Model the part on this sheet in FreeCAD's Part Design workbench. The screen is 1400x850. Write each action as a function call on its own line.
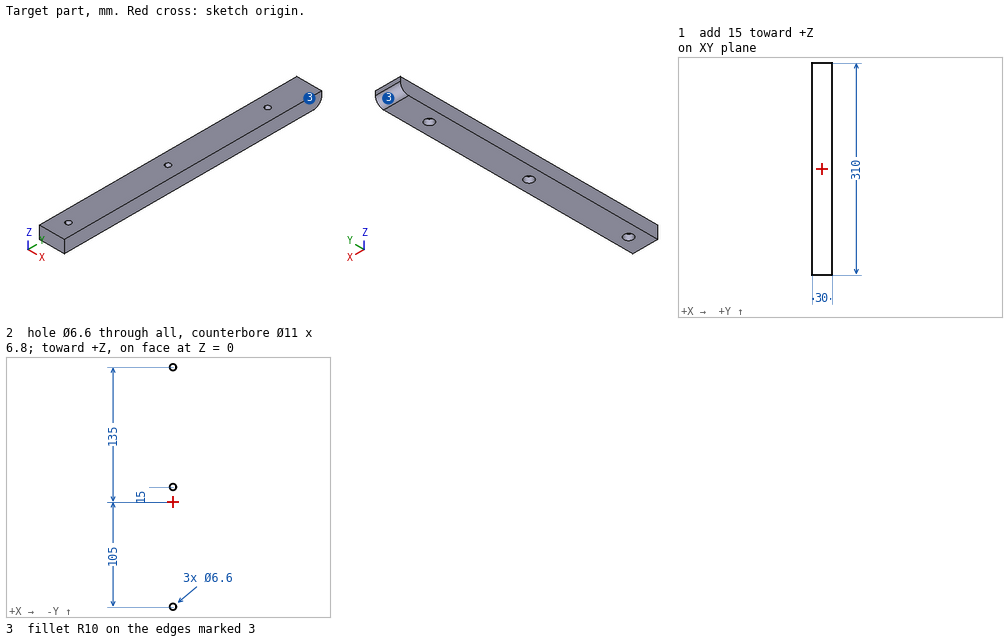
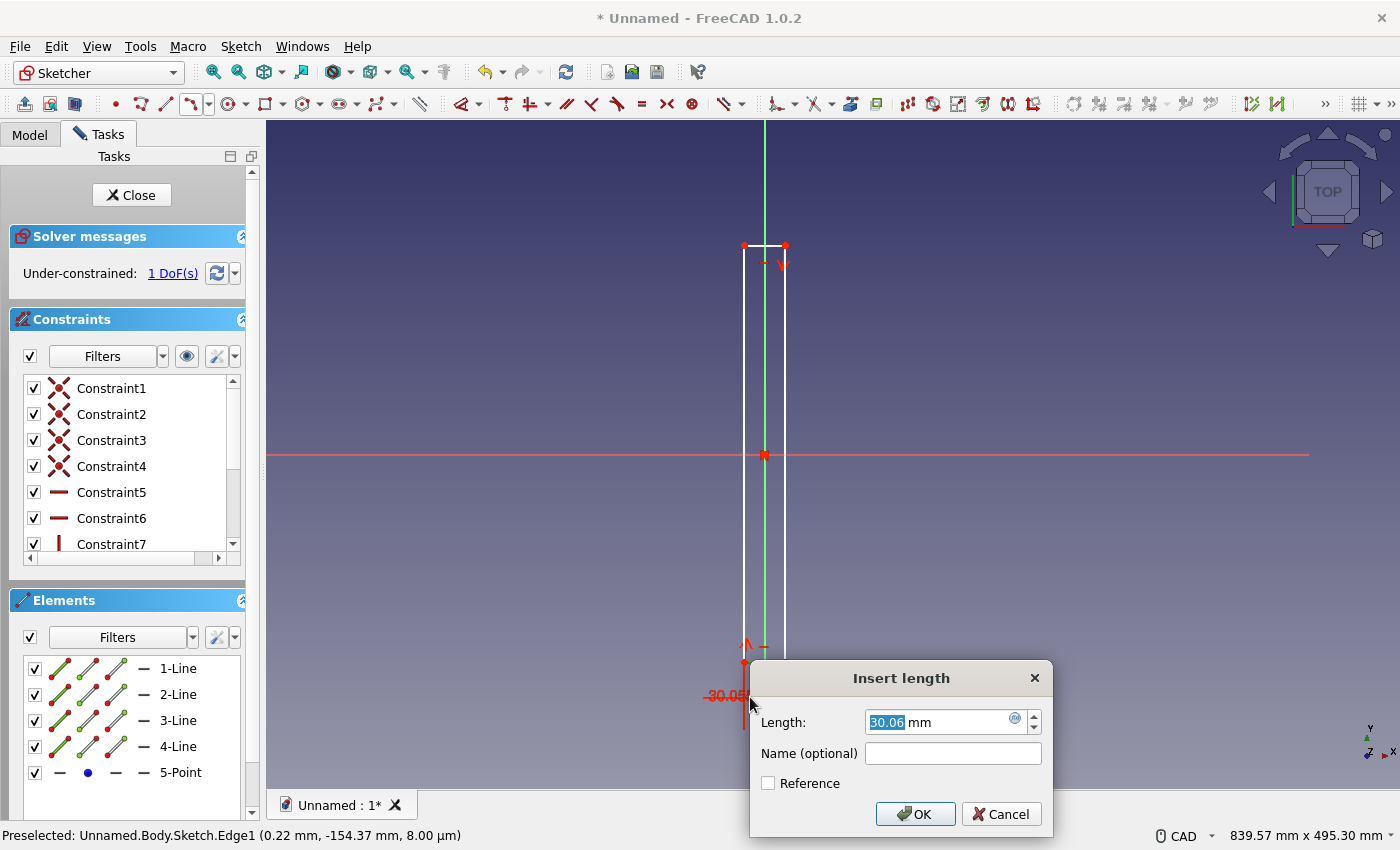
text(30)
key(Return)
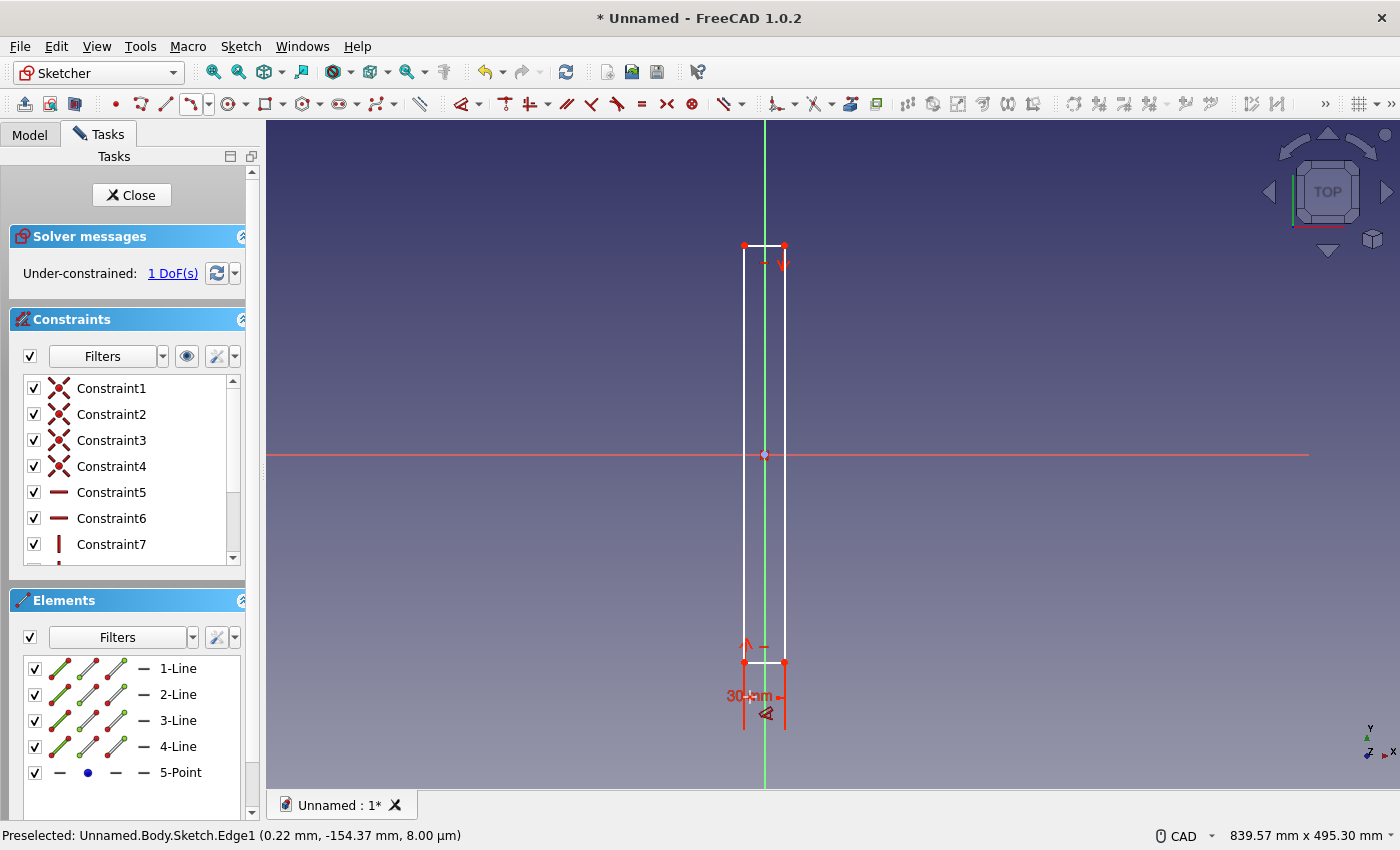
click(785, 538)
click(819, 359)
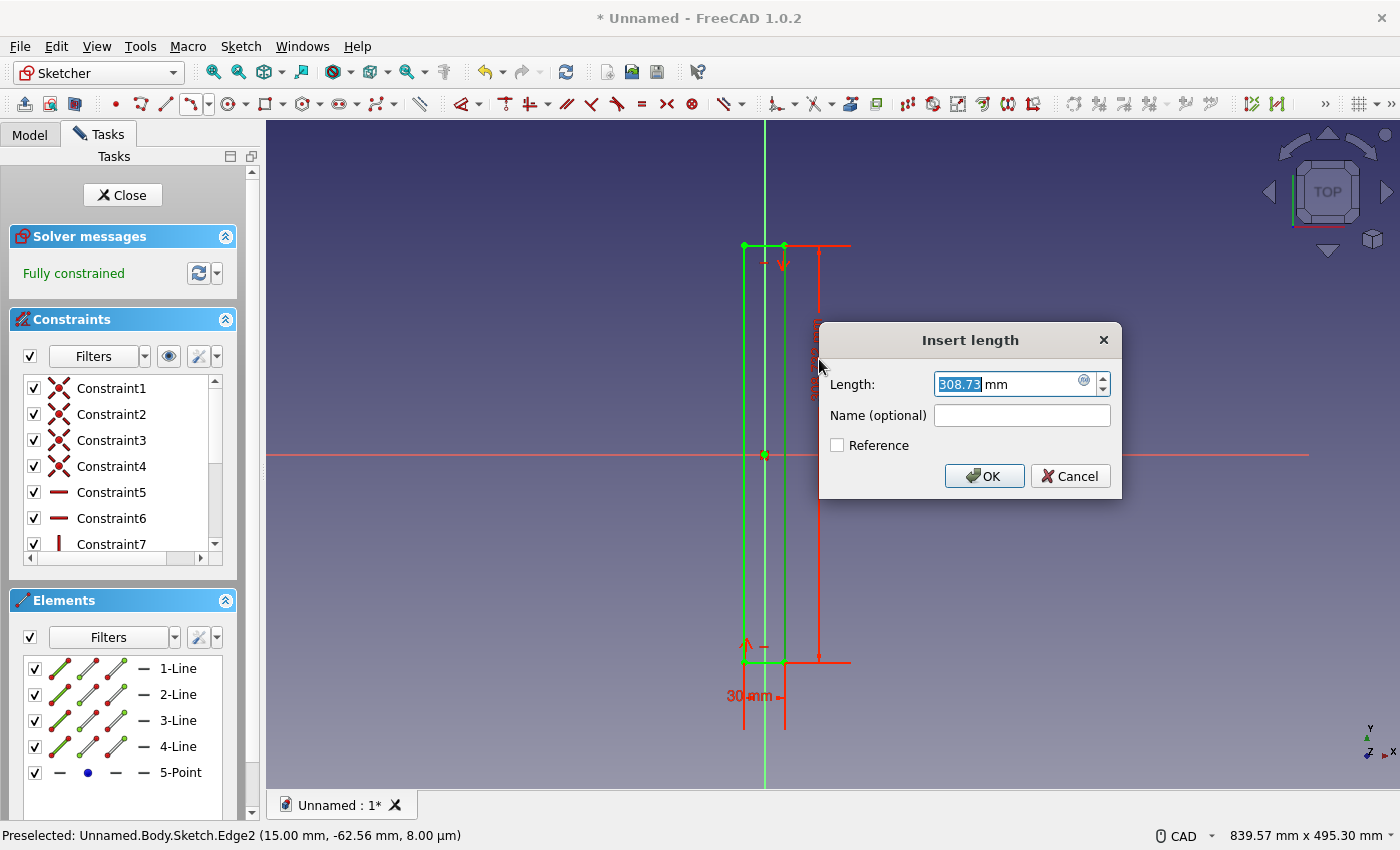
text(310)
key(Return)
key(Escape)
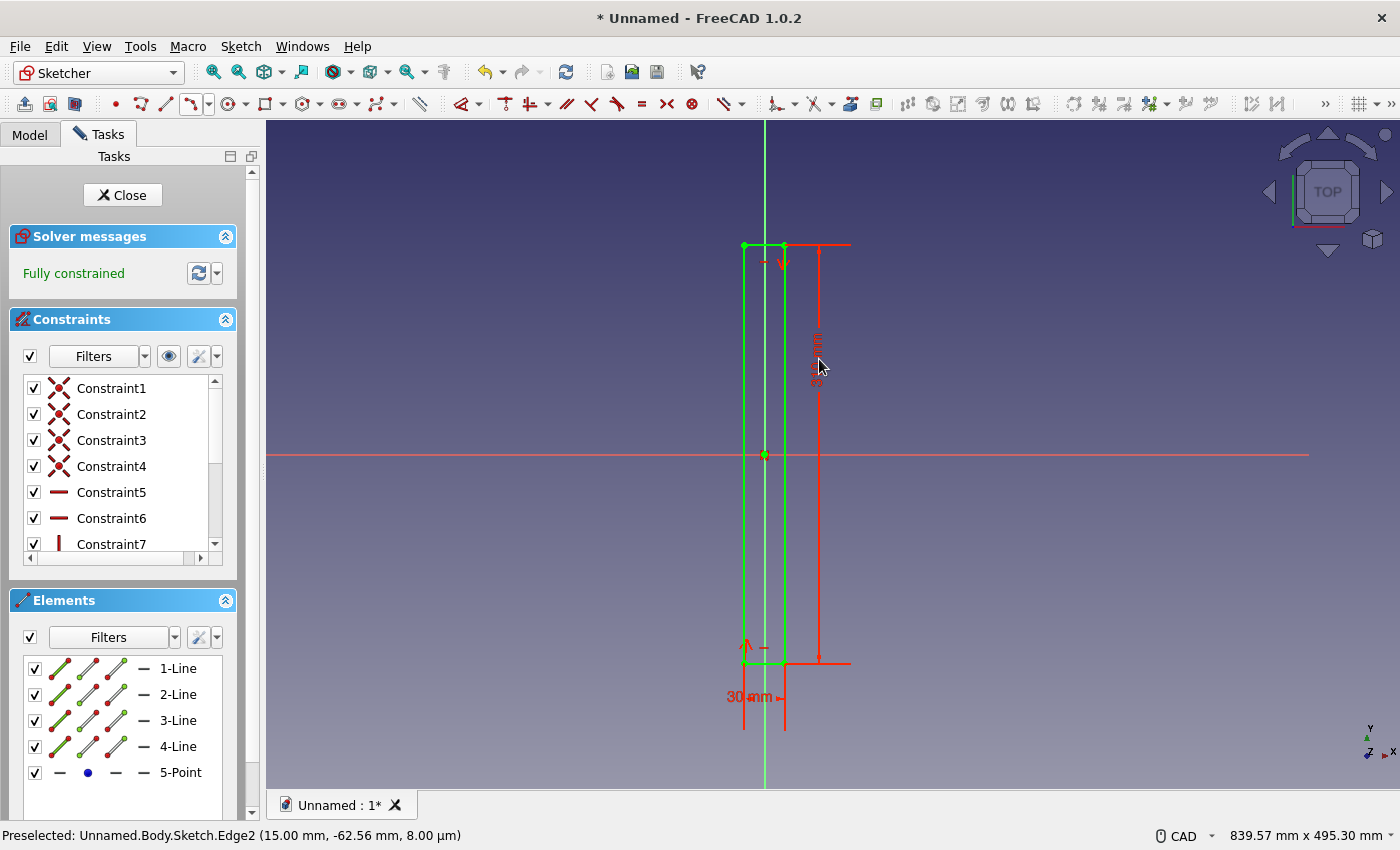
click(123, 195)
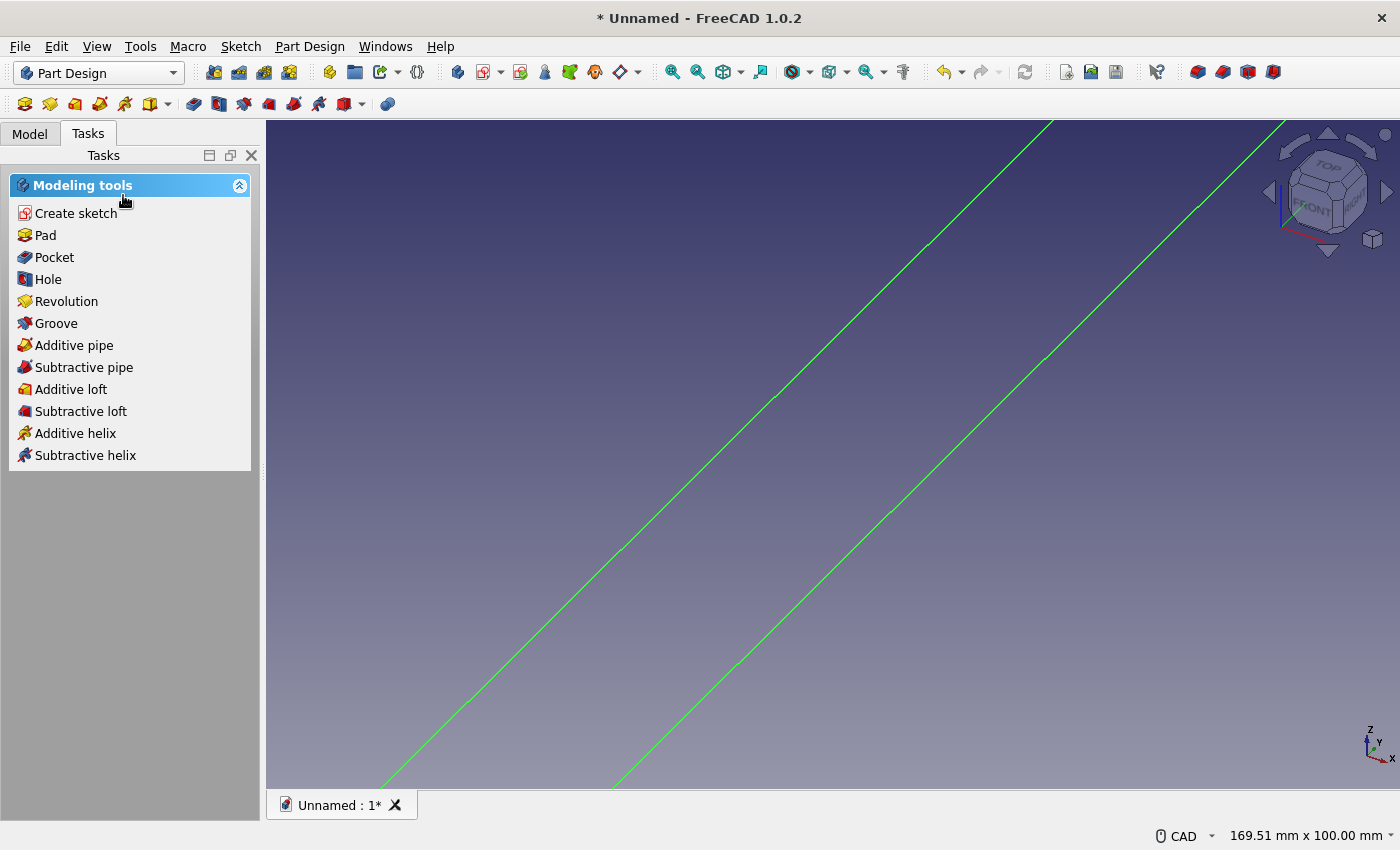
click(25, 104)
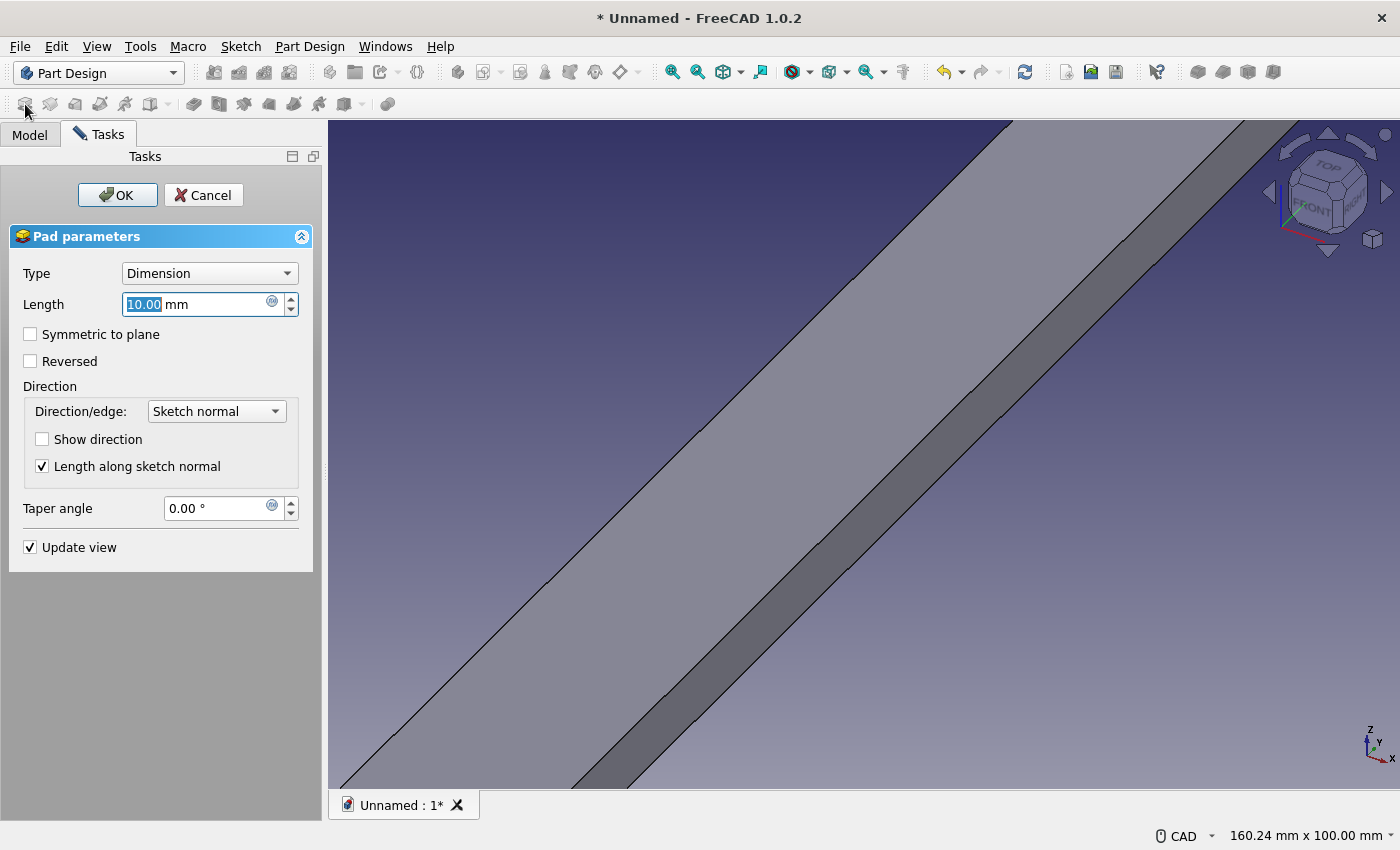
text(15)
key(Tab)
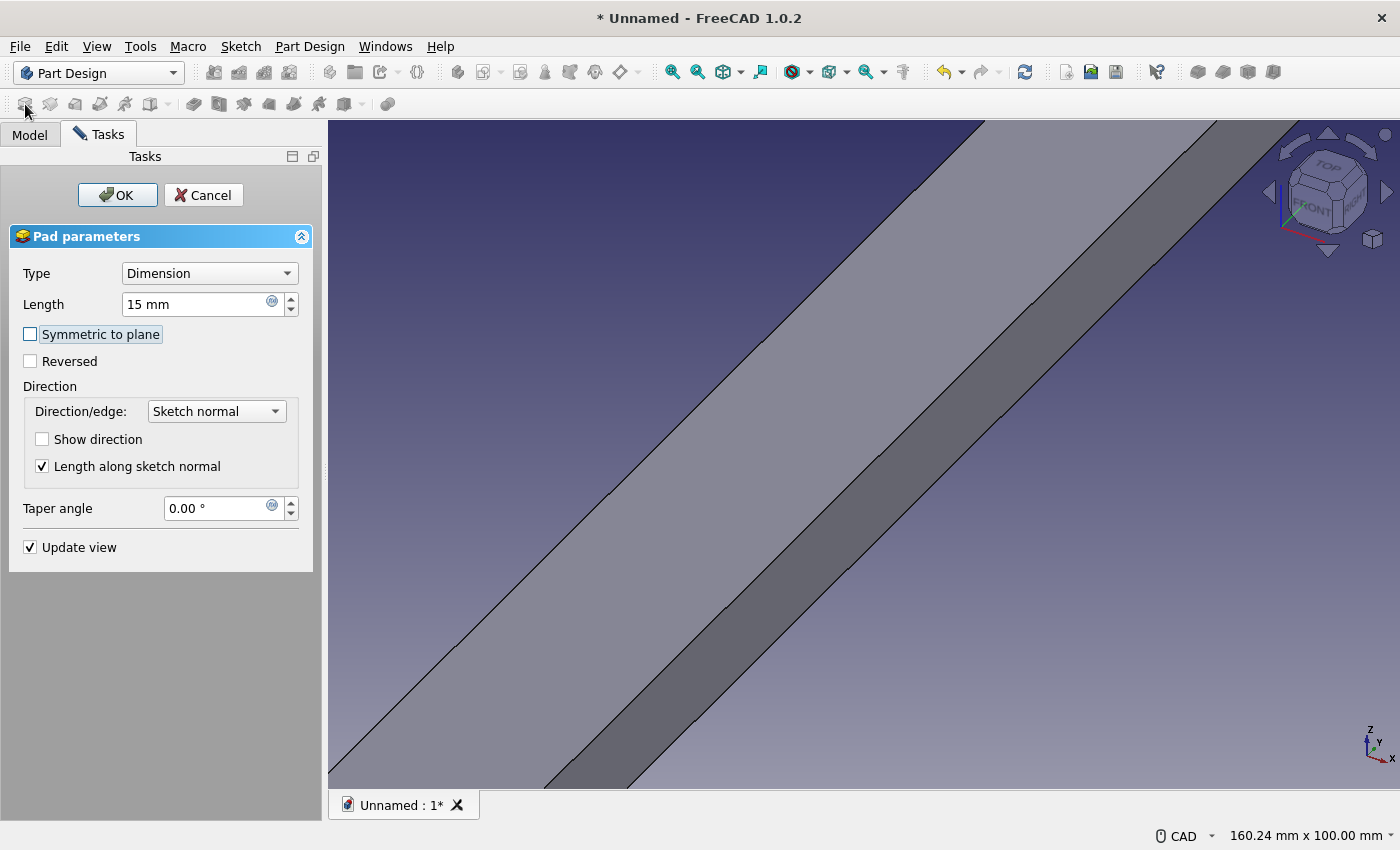
click(118, 195)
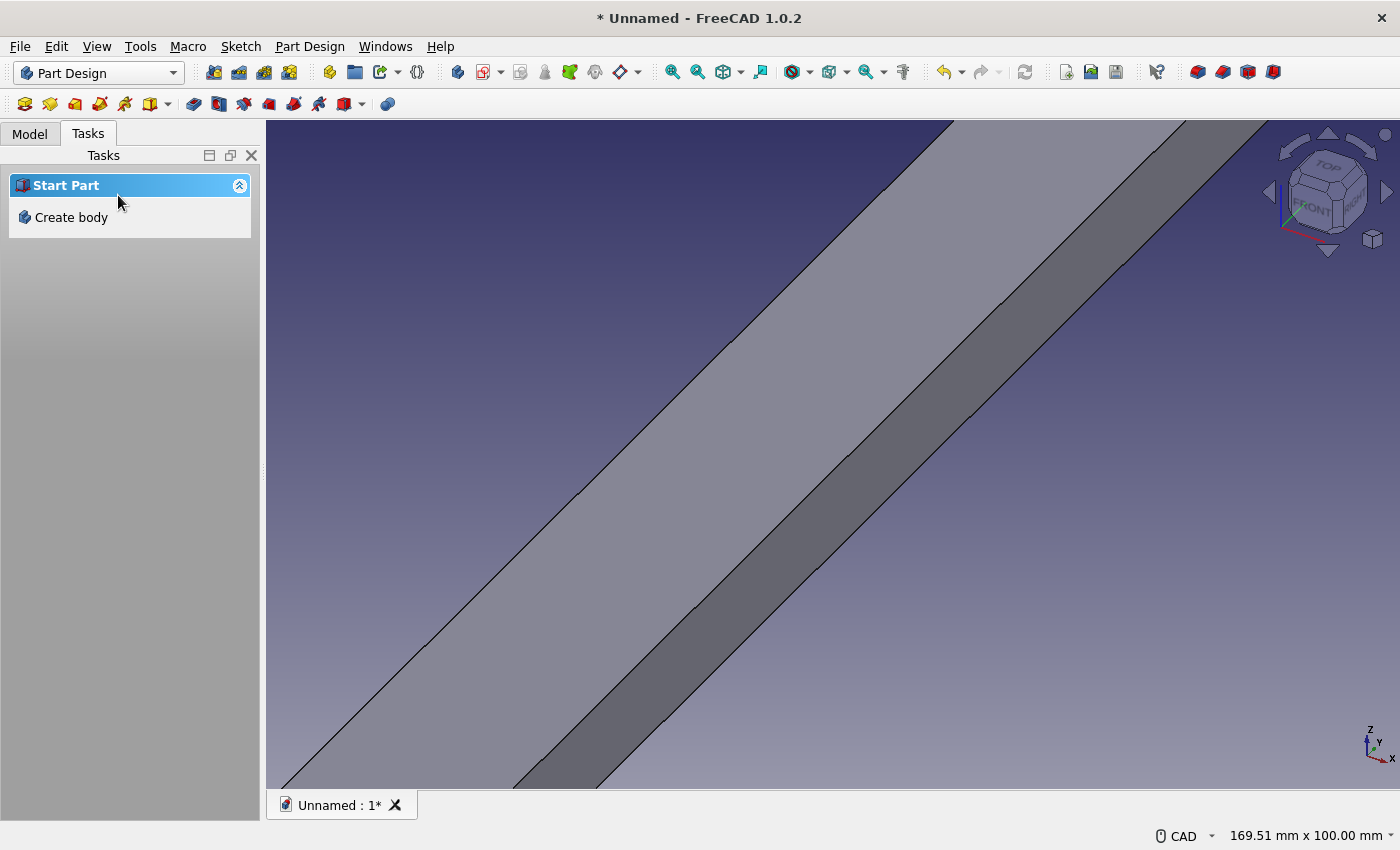
click(673, 72)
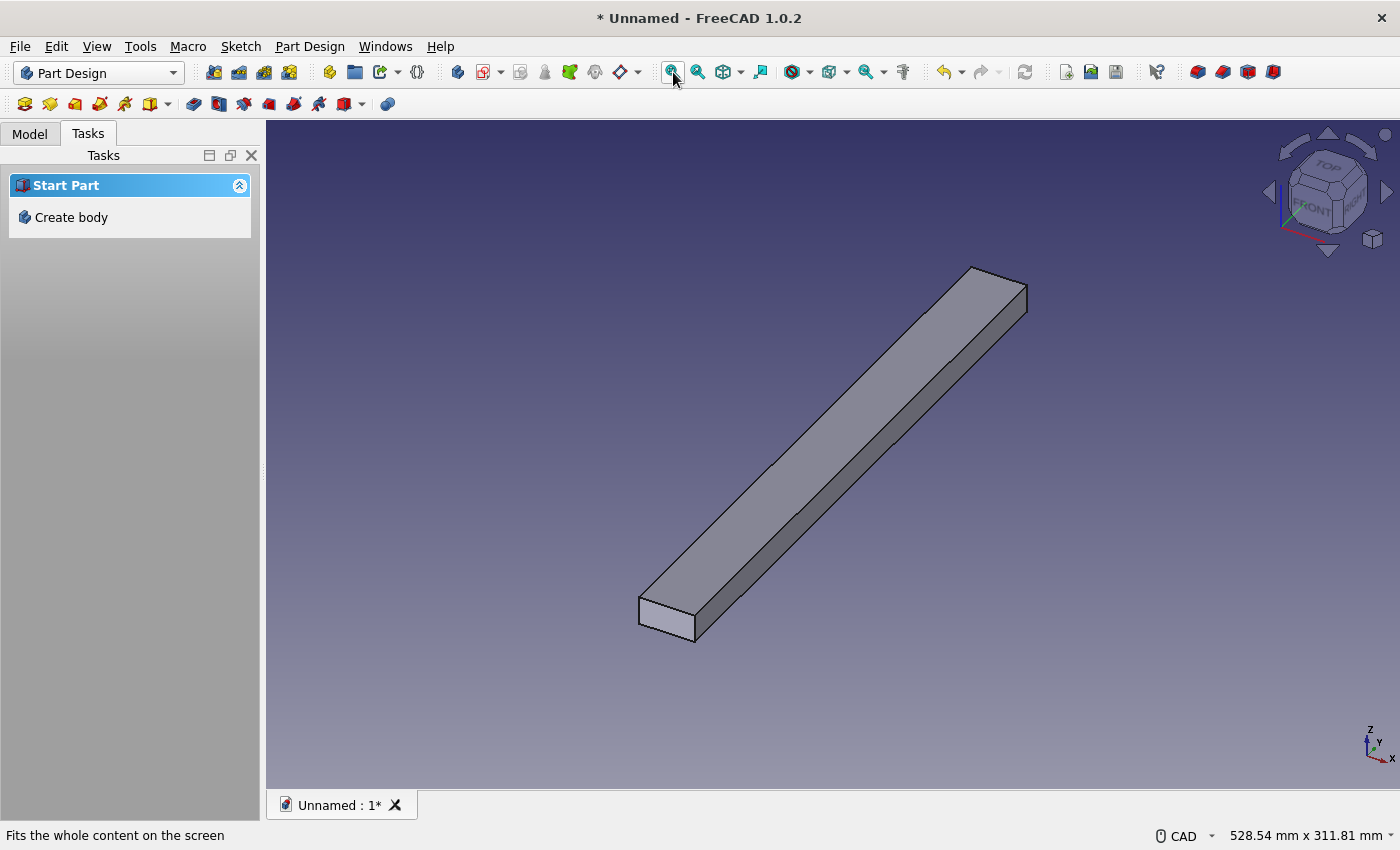
key(5)